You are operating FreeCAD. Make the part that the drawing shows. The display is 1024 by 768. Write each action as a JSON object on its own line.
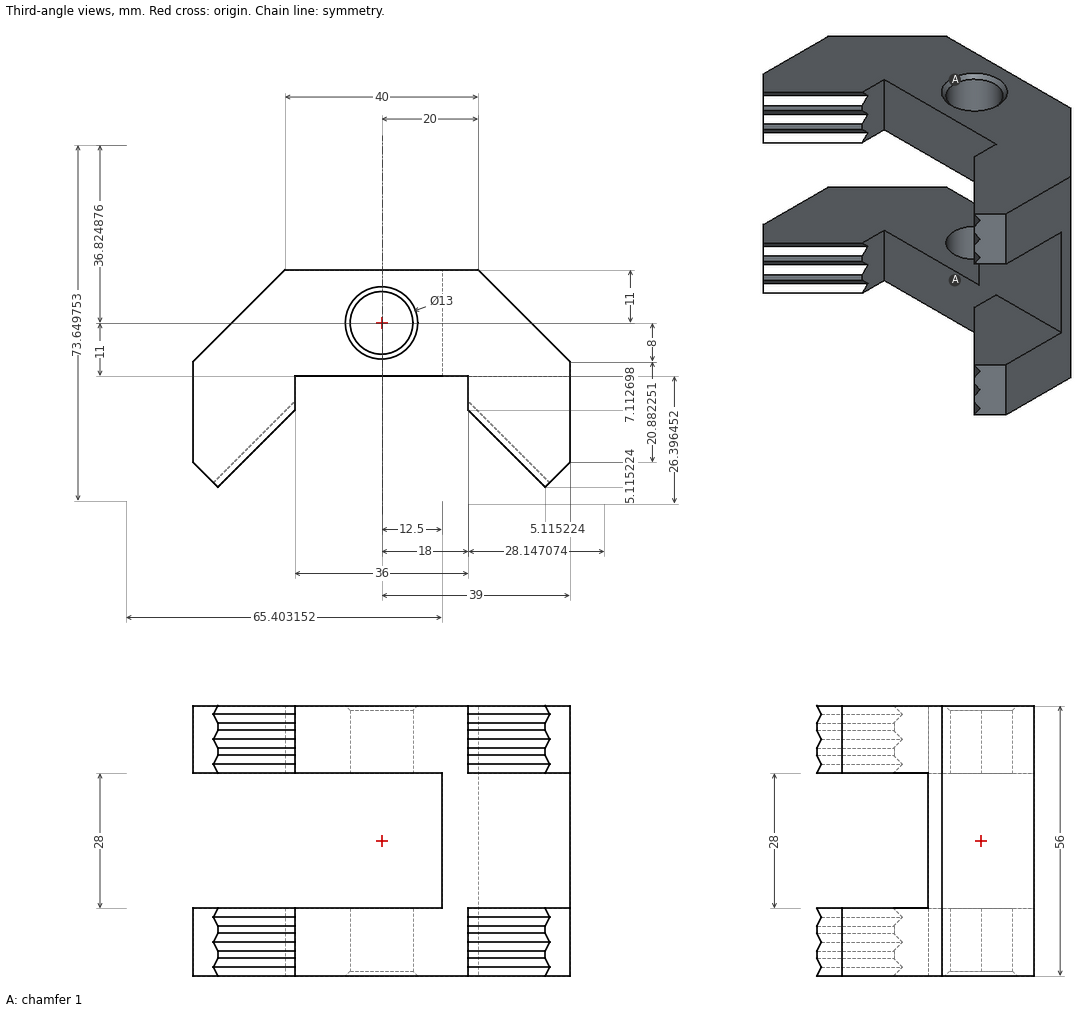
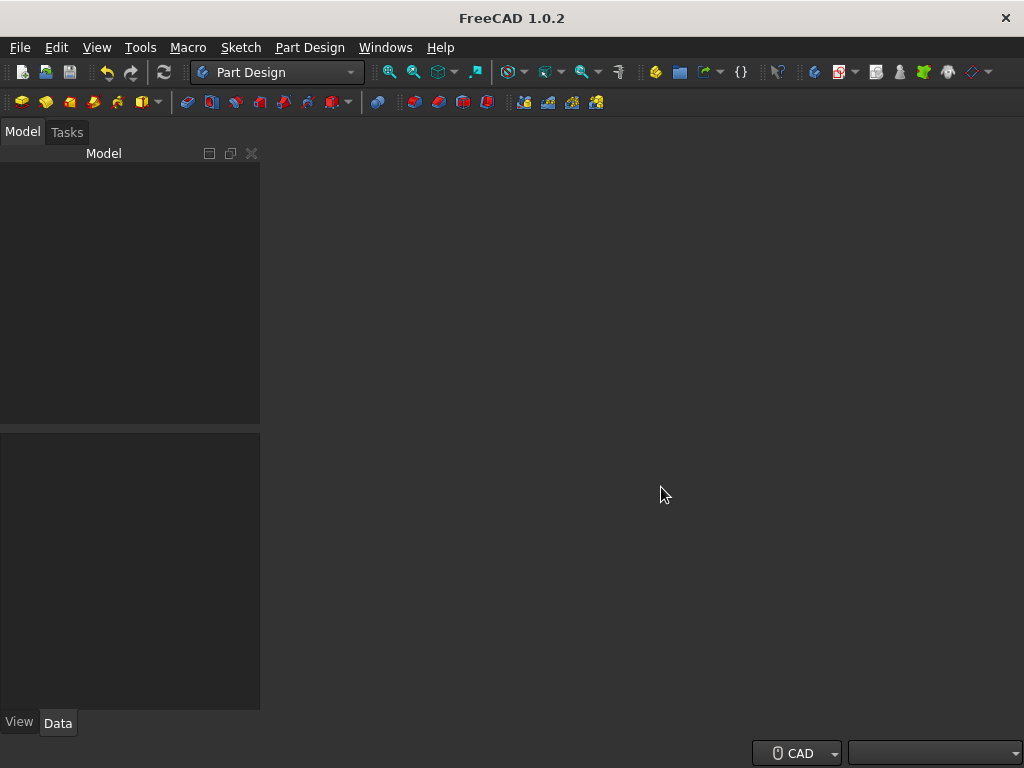
{"action": "left_click", "coordinate": [22, 72]}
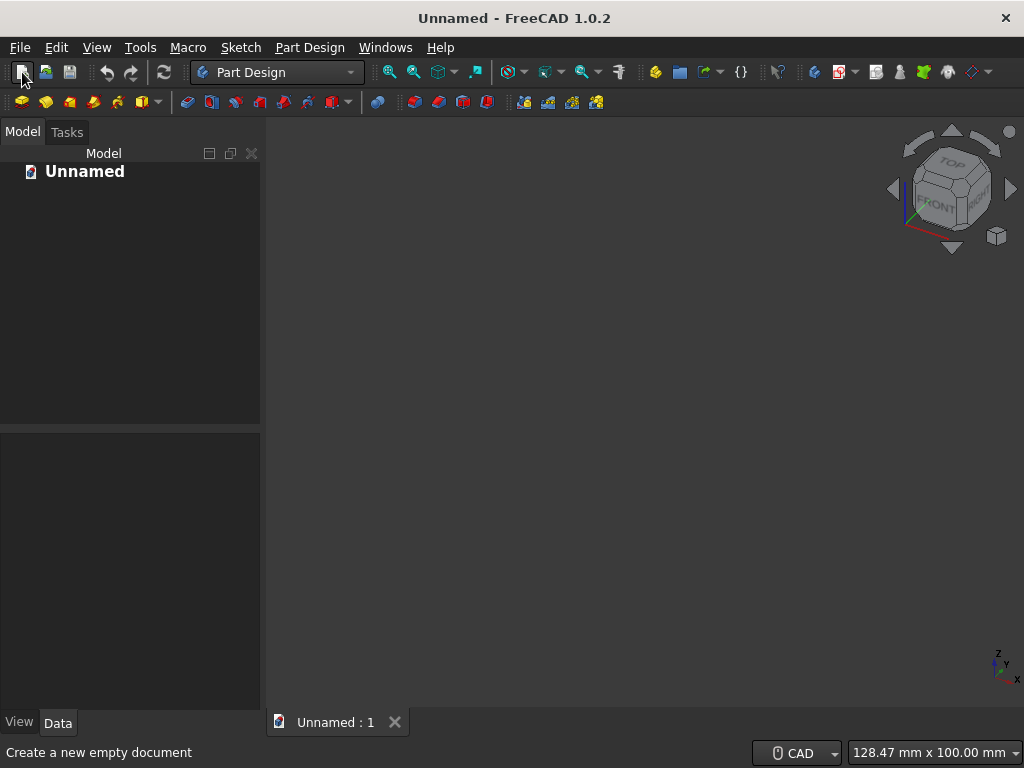
{"action": "left_click", "coordinate": [840, 72]}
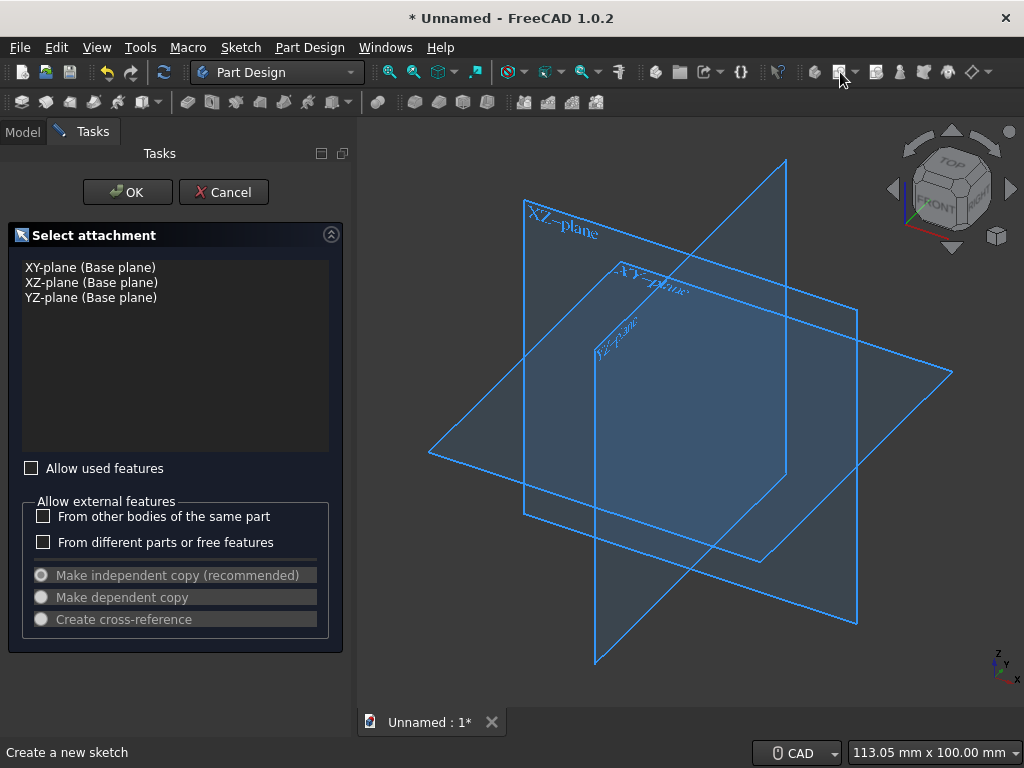
{"action": "left_click", "coordinate": [82, 268]}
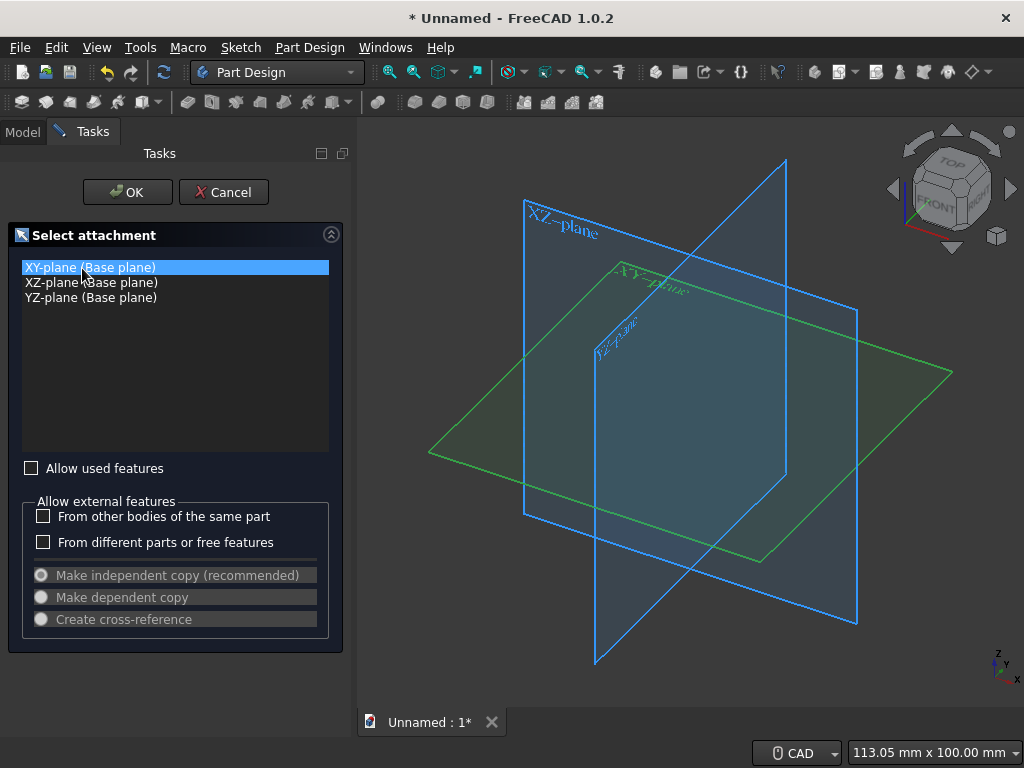
{"action": "left_click", "coordinate": [128, 192]}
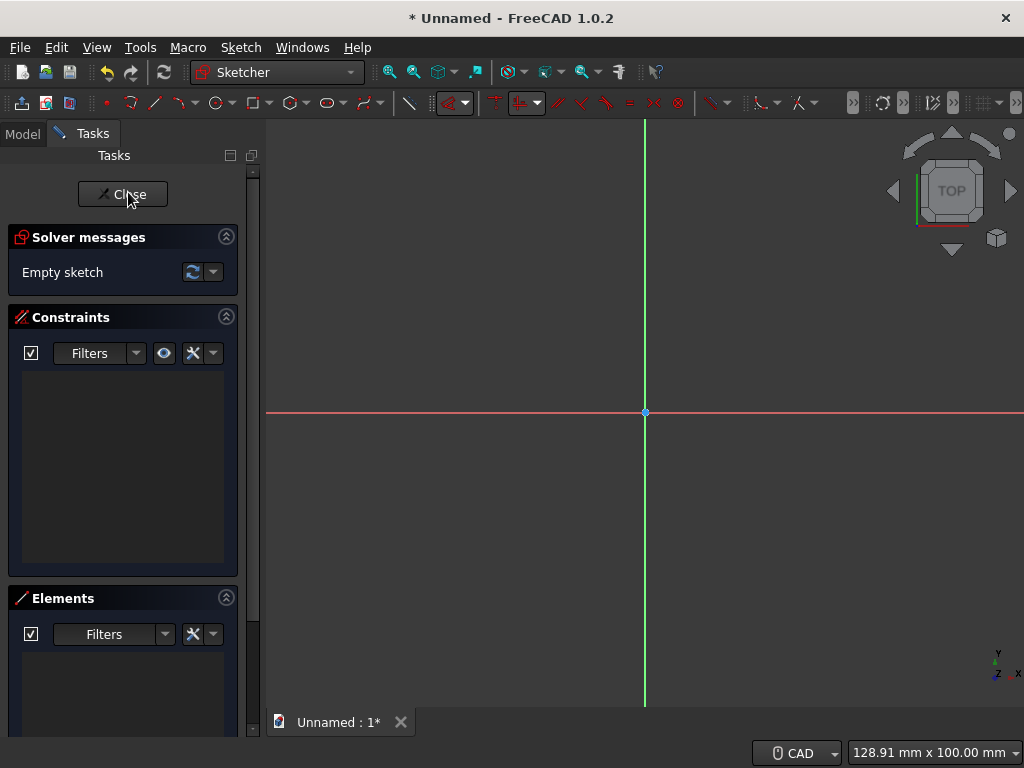
{"action": "scroll", "coordinate": [294, 147], "scroll_direction": "down", "scroll_amount": 1}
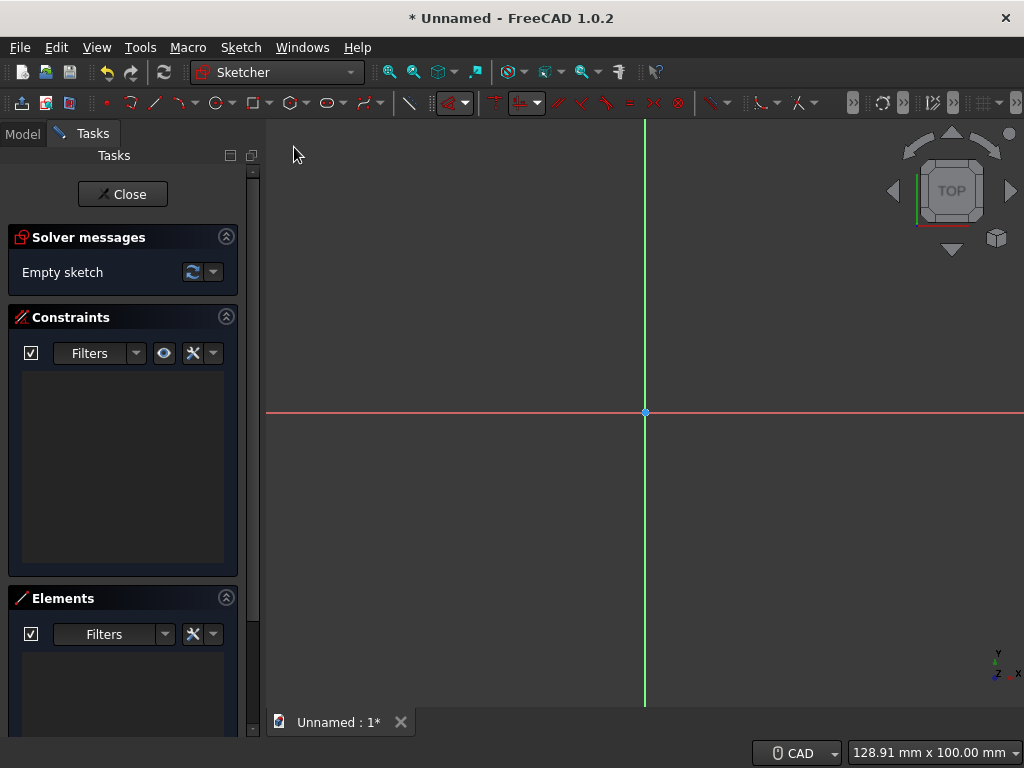
{"action": "left_click", "coordinate": [132, 104]}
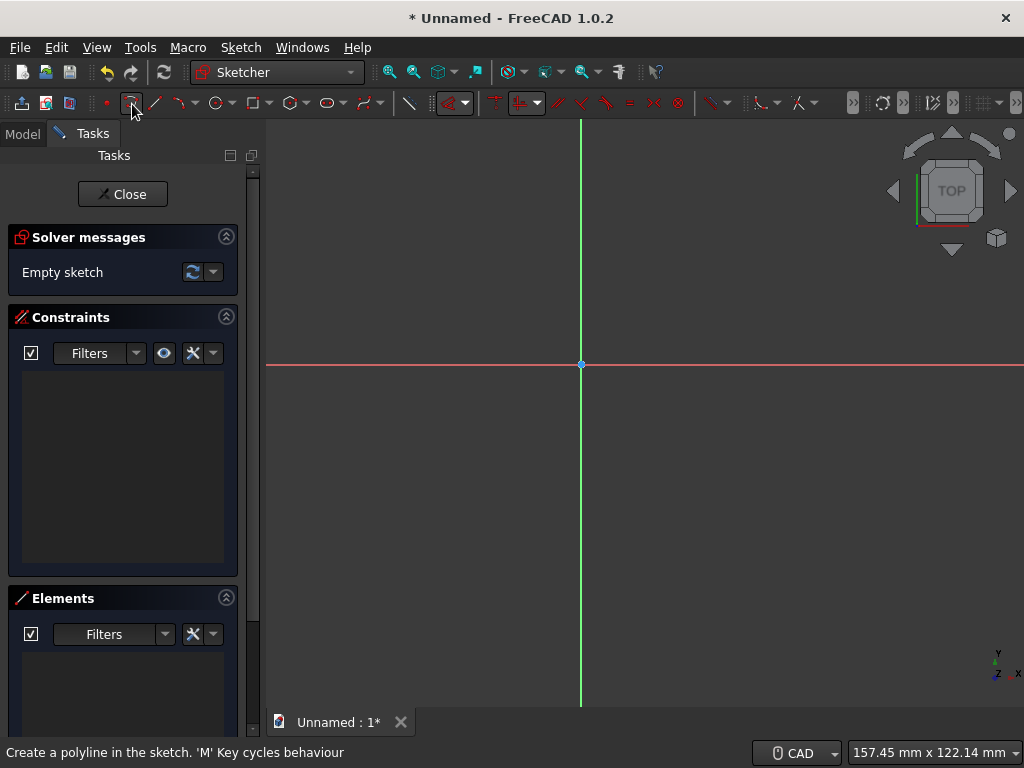
{"action": "left_click", "coordinate": [495, 418]}
{"action": "left_click", "coordinate": [668, 418]}
{"action": "left_click", "coordinate": [668, 452]}
{"action": "left_click", "coordinate": [745, 528]}
{"action": "left_click", "coordinate": [769, 504]}
{"action": "left_click", "coordinate": [769, 403]}
{"action": "left_click", "coordinate": [678, 312]}
{"action": "left_click", "coordinate": [485, 312]}
{"action": "left_click", "coordinate": [394, 403]}
{"action": "left_click", "coordinate": [394, 504]}
{"action": "left_click", "coordinate": [418, 528]}
{"action": "left_click", "coordinate": [495, 452]}
{"action": "left_click", "coordinate": [495, 419]}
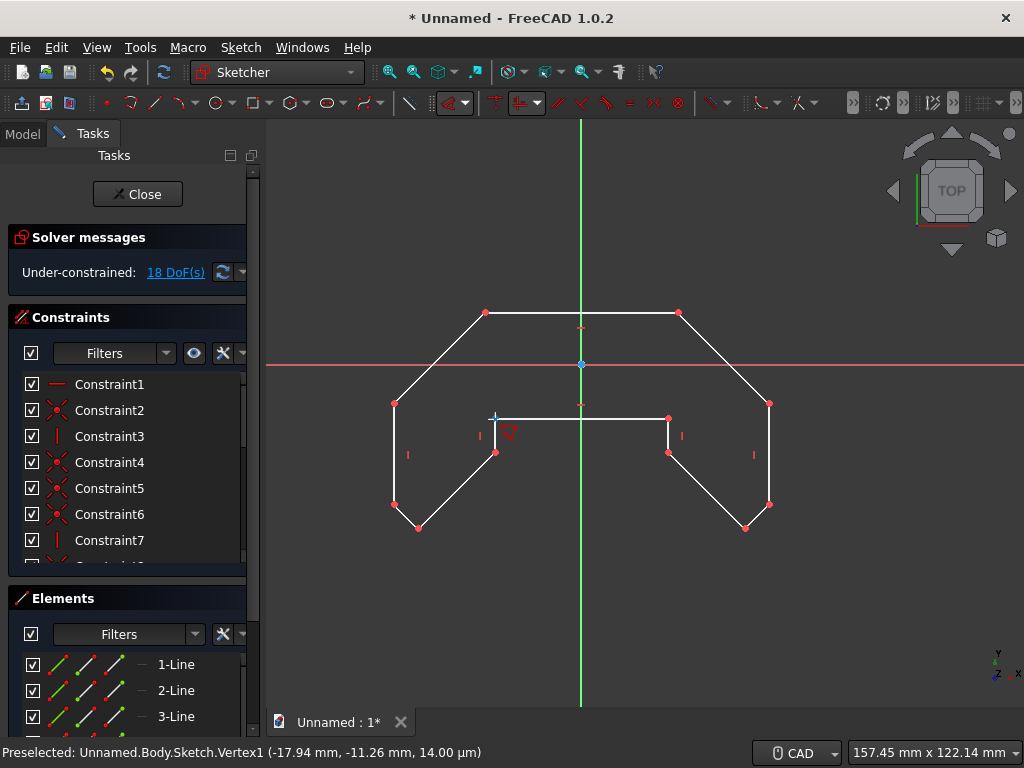
{"action": "left_click", "coordinate": [216, 104]}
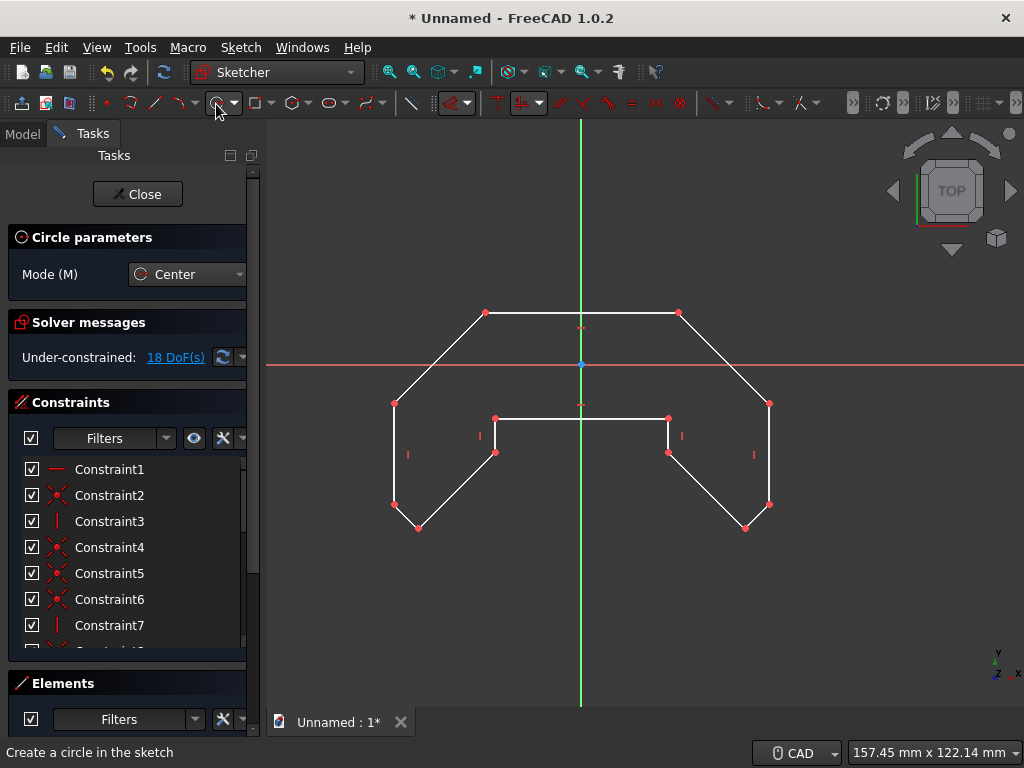
{"action": "left_click", "coordinate": [581, 365]}
{"action": "left_click", "coordinate": [604, 343]}
{"action": "key", "text": "Escape"}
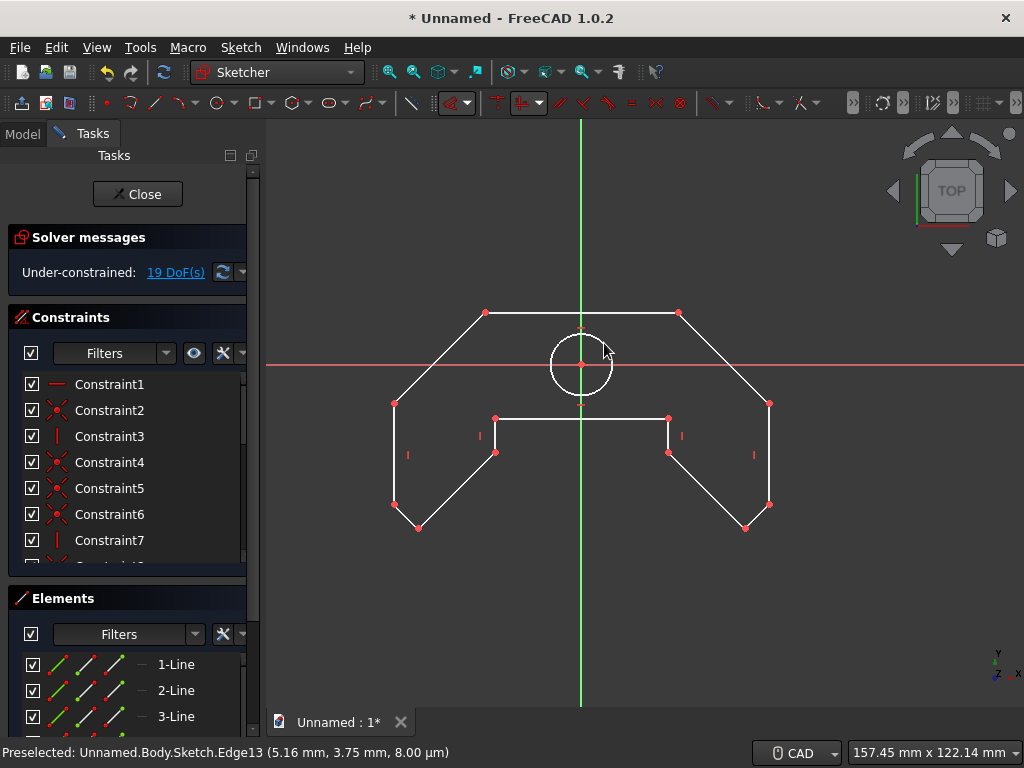
{"action": "left_click", "coordinate": [769, 404]}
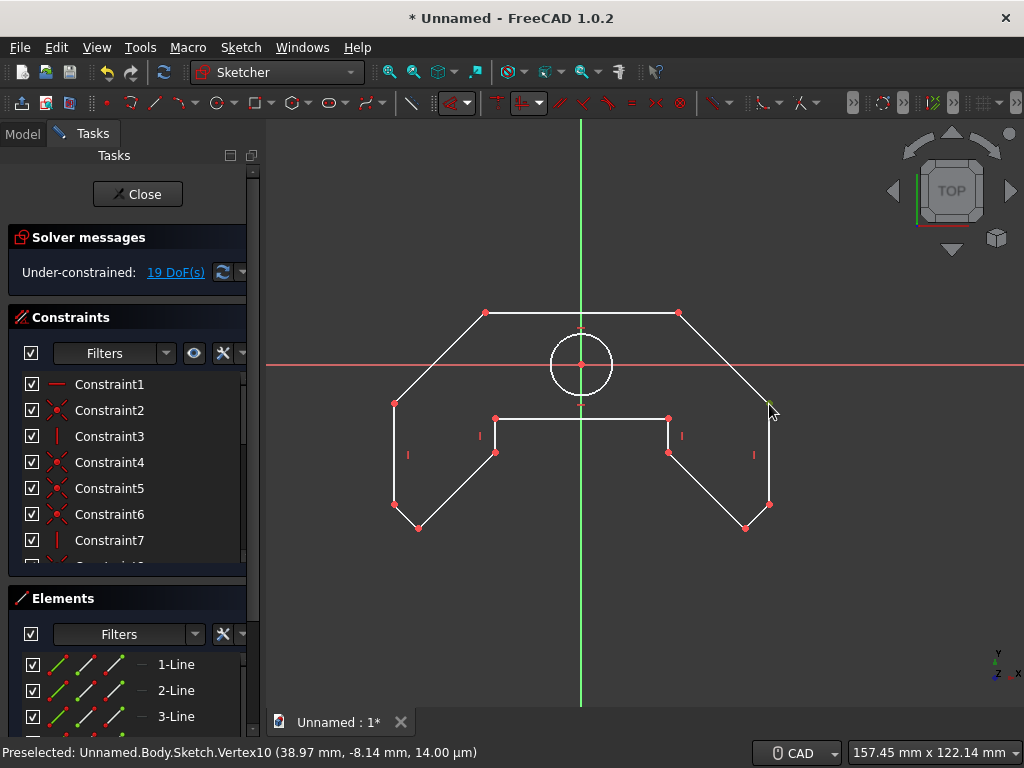
{"action": "left_click", "coordinate": [394, 404]}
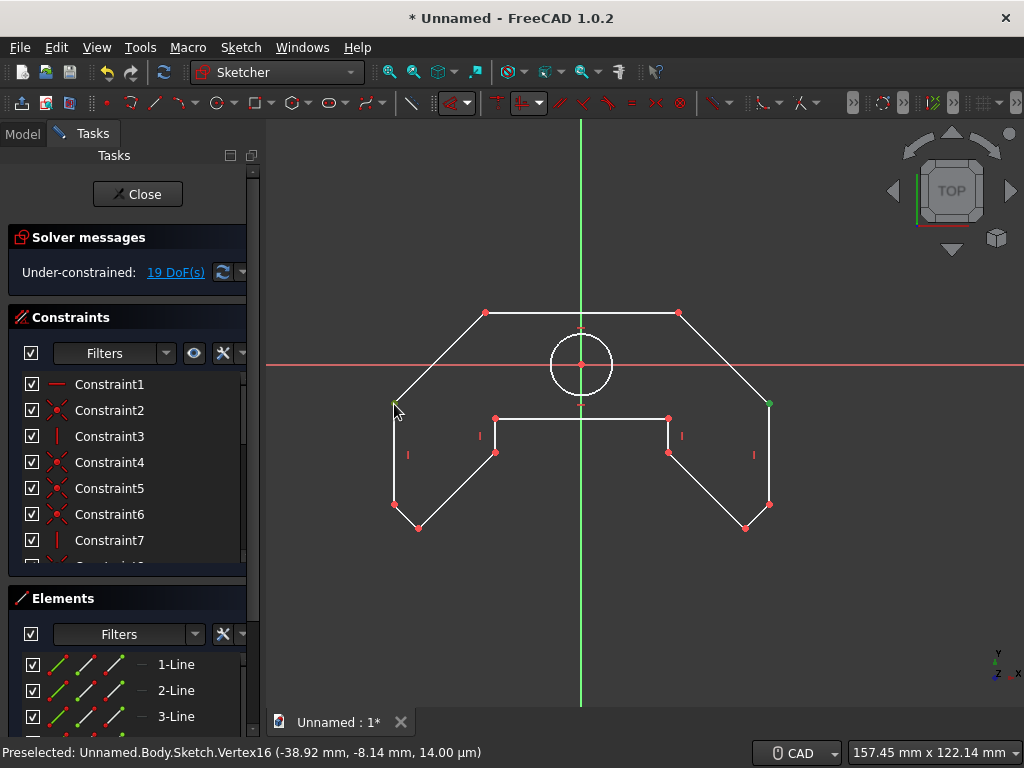
{"action": "left_click", "coordinate": [581, 641]}